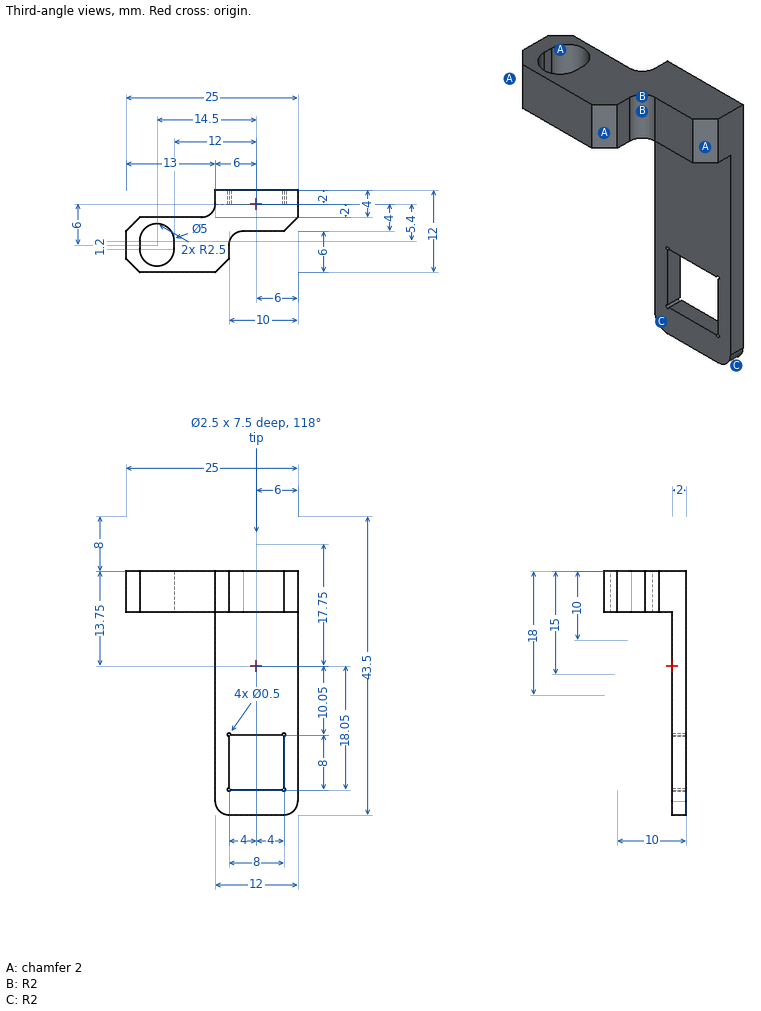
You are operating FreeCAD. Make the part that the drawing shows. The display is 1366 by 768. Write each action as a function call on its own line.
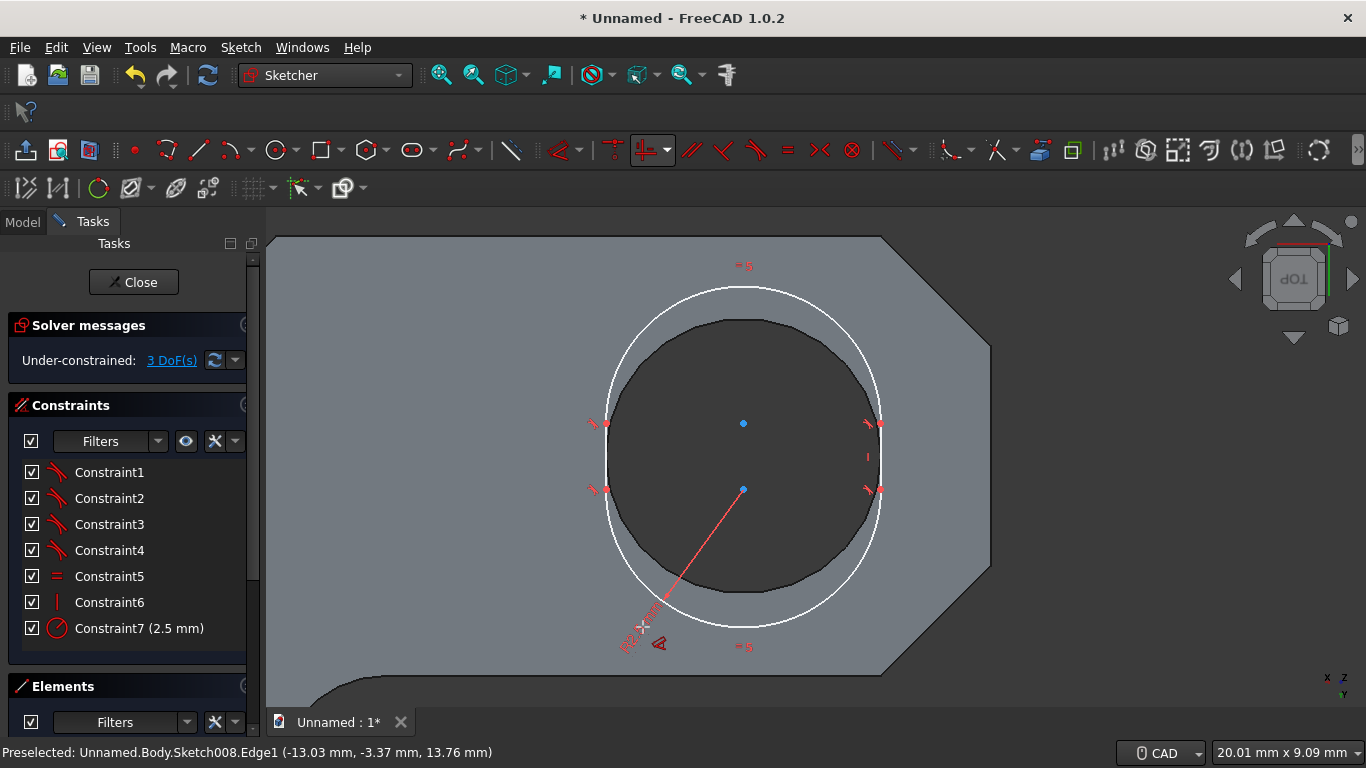
click(606, 470)
click(572, 457)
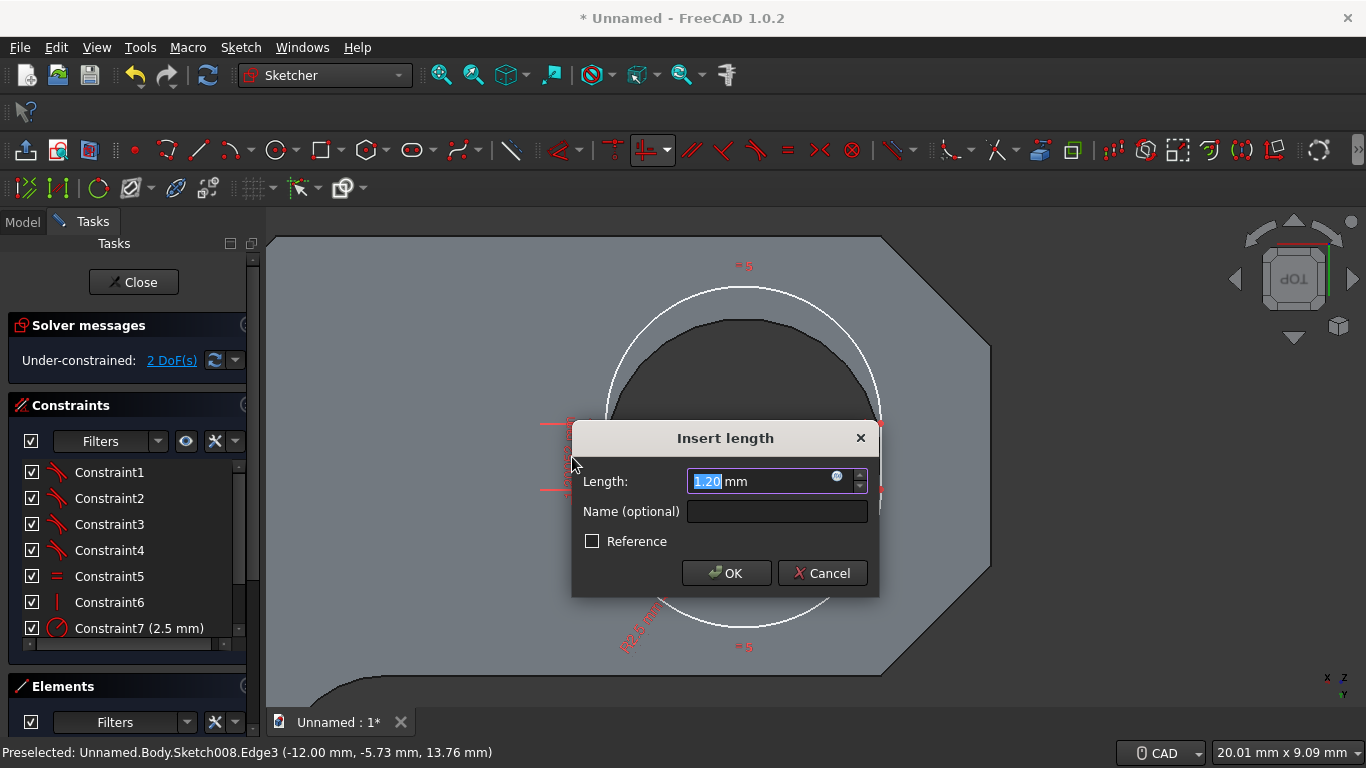
text(1.2)
key(Return)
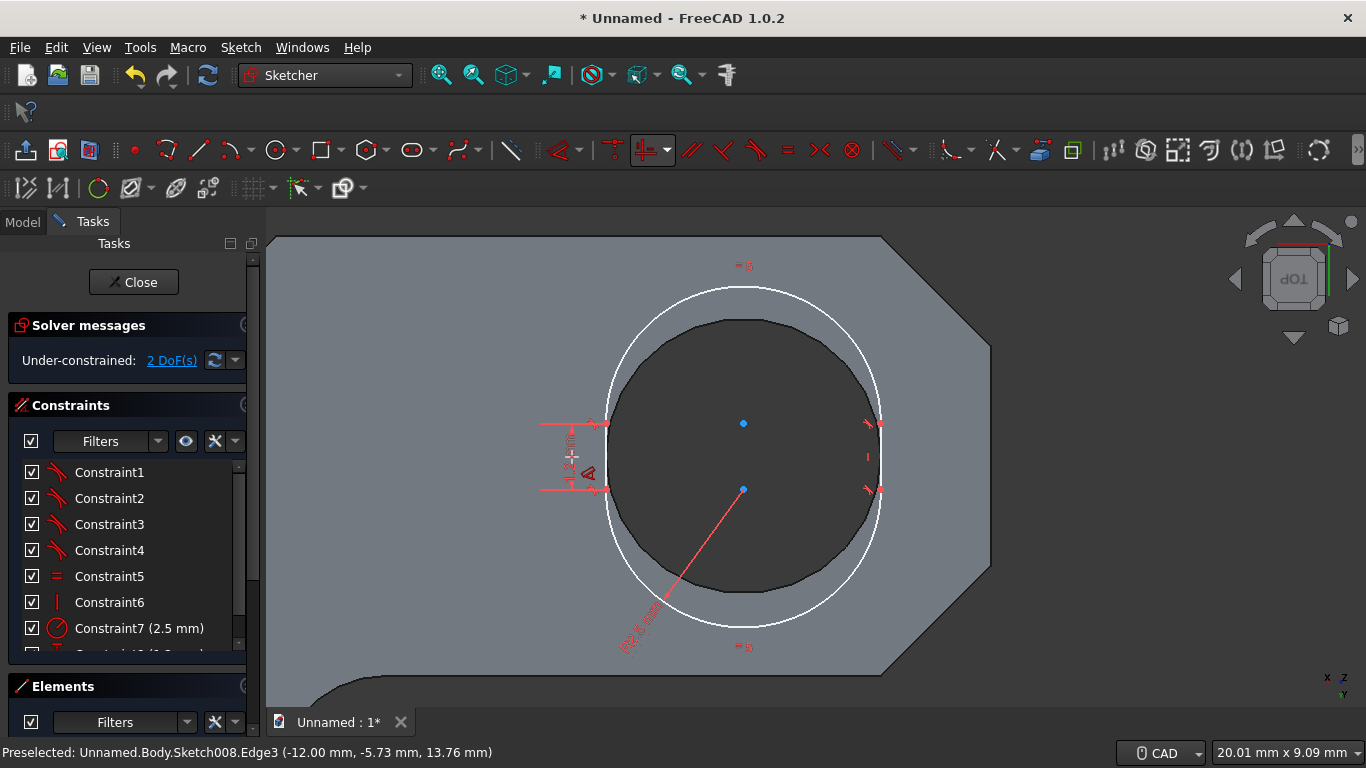
click(606, 490)
click(450, 456)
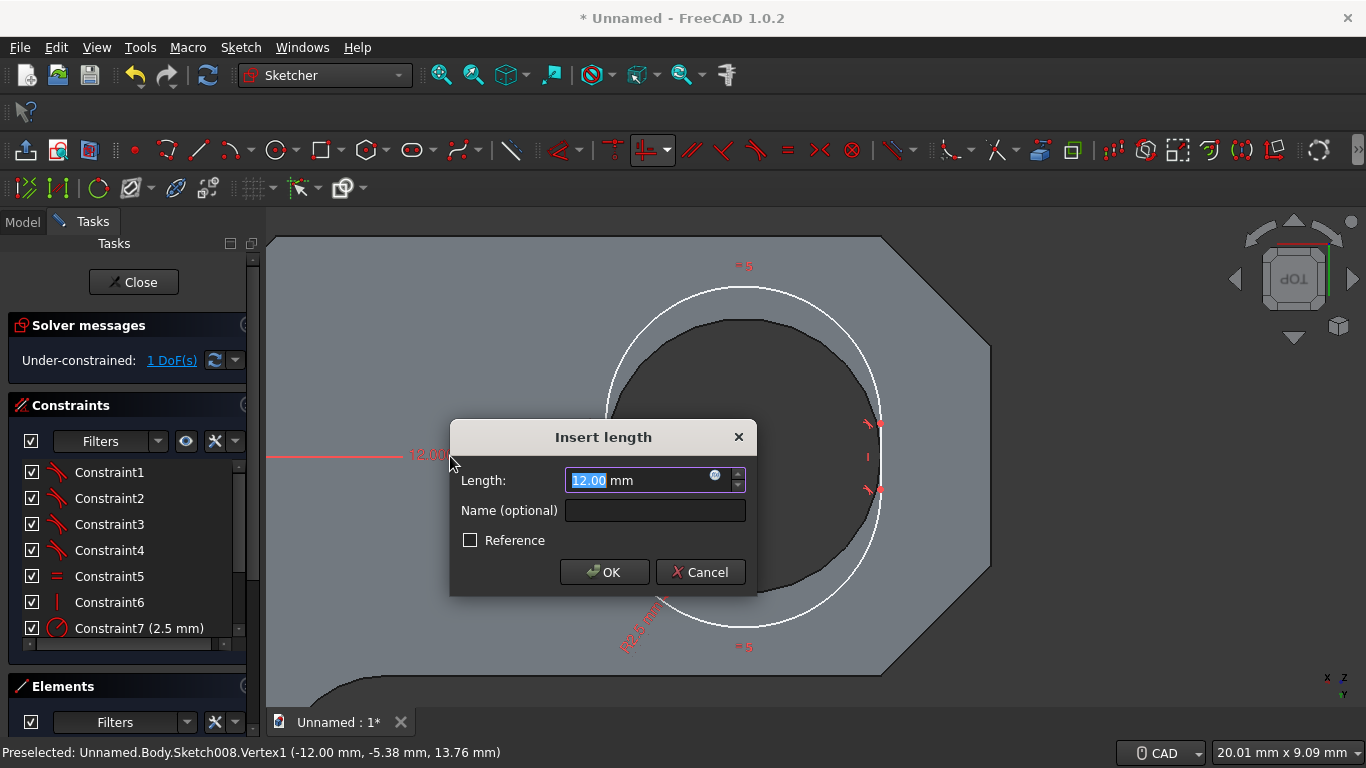
text(12)
key(Return)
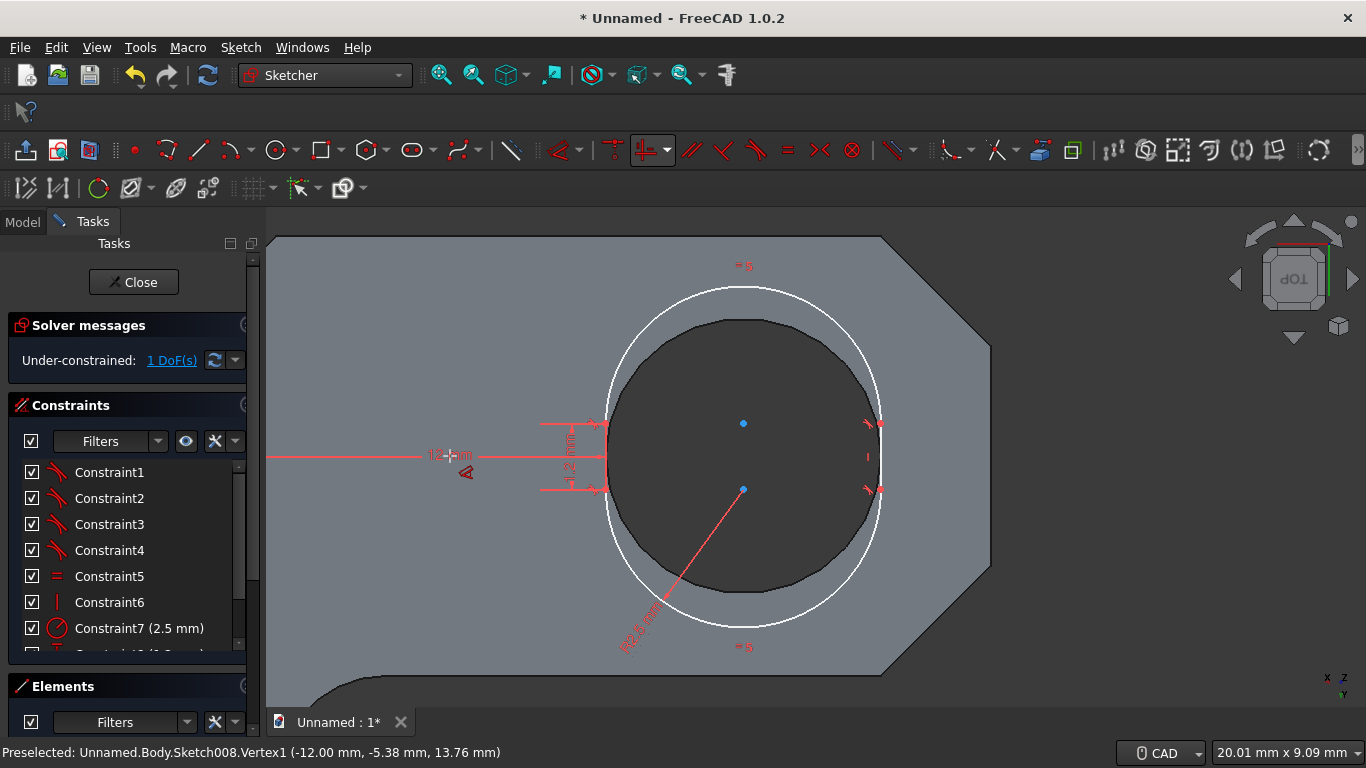
click(606, 490)
click(640, 541)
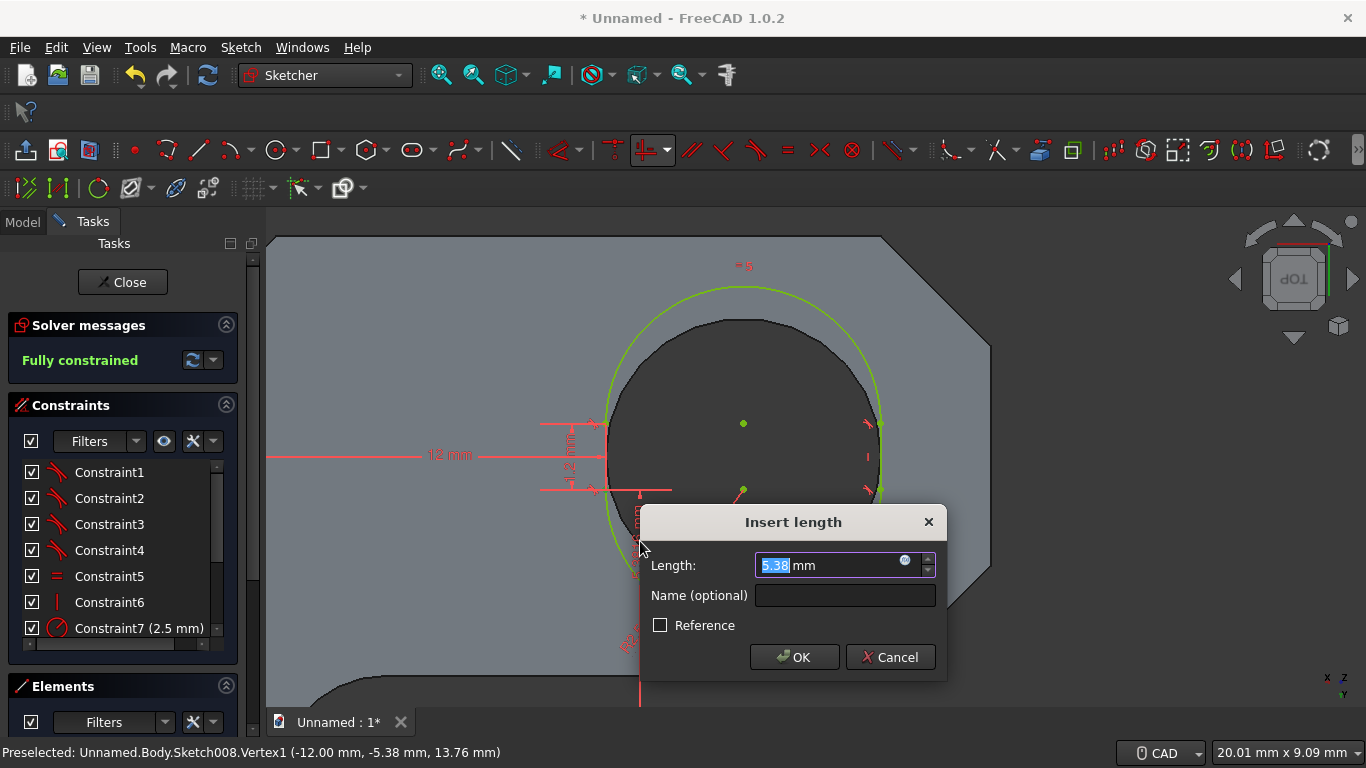
text(5.4)
key(Return)
key(Escape)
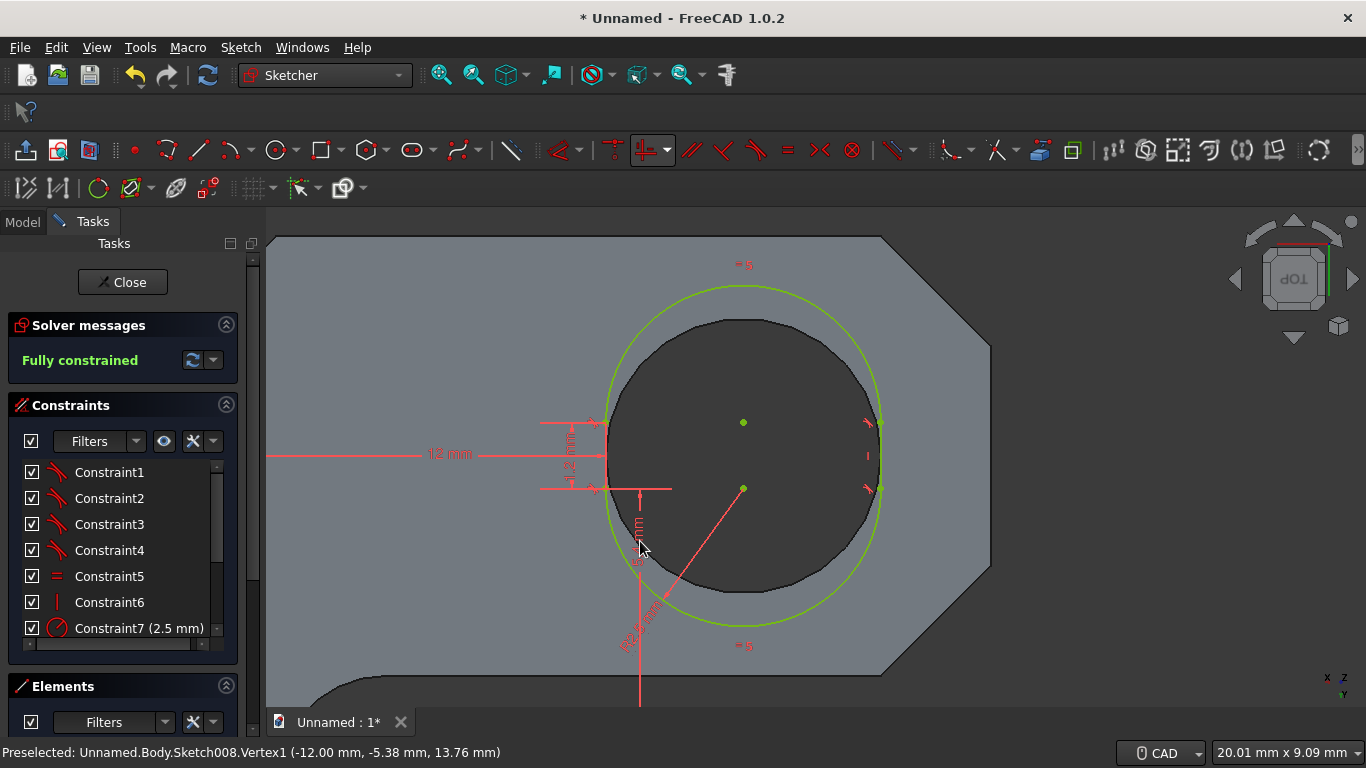
click(123, 282)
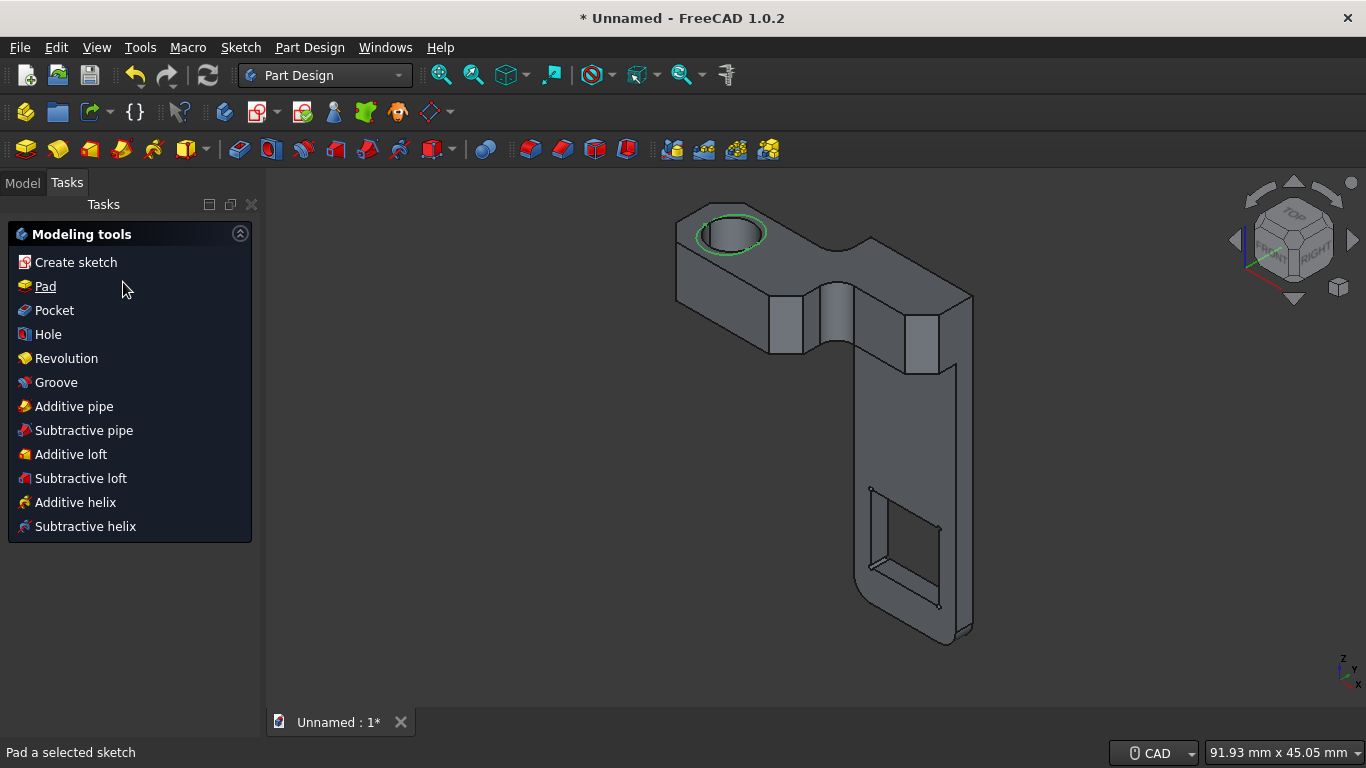
click(240, 150)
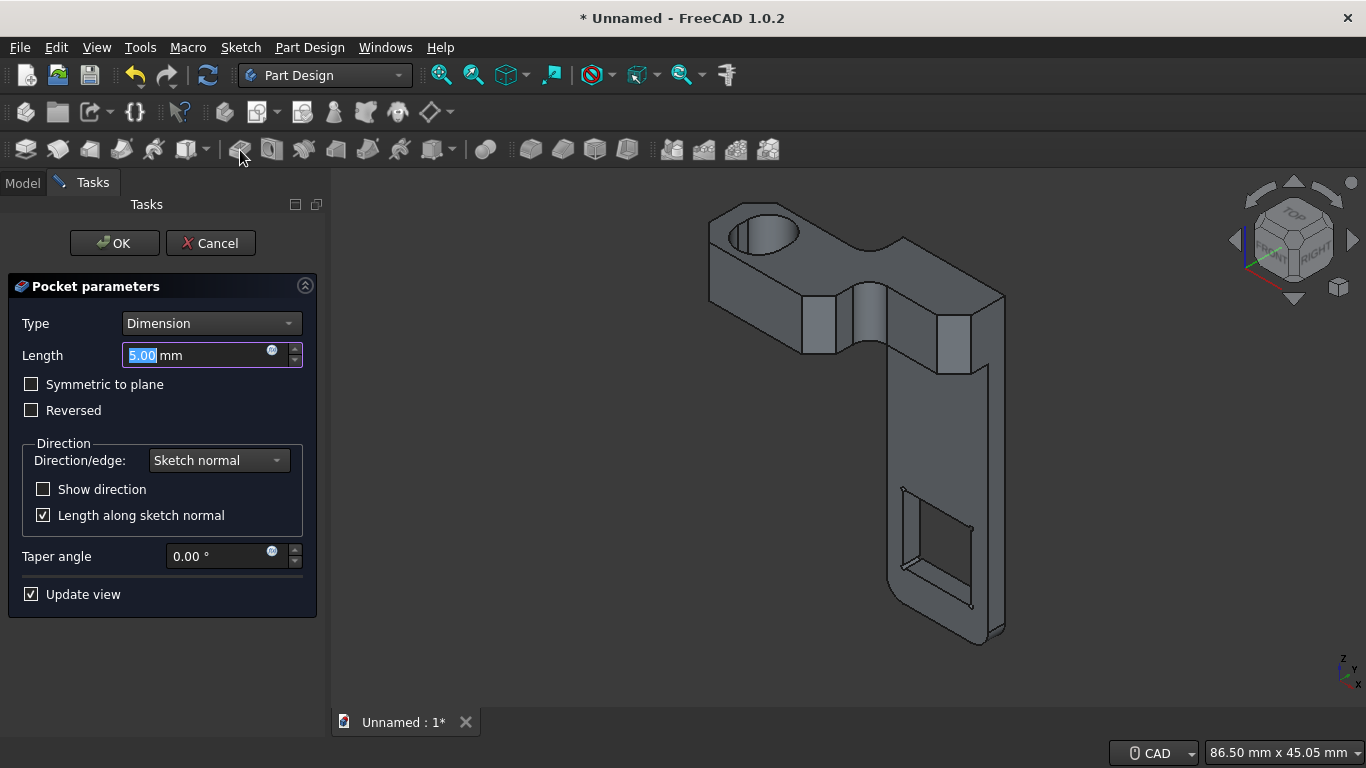
text(10)
key(Tab)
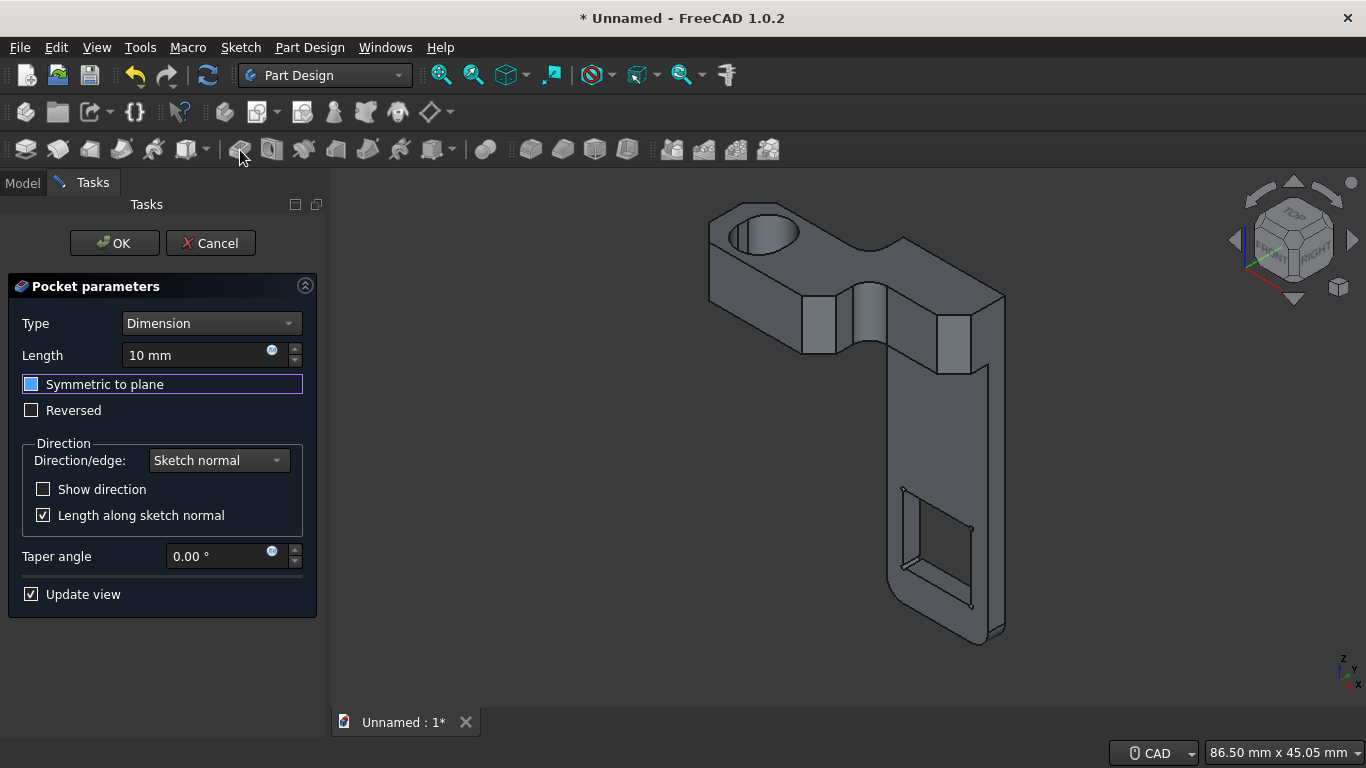
click(115, 243)